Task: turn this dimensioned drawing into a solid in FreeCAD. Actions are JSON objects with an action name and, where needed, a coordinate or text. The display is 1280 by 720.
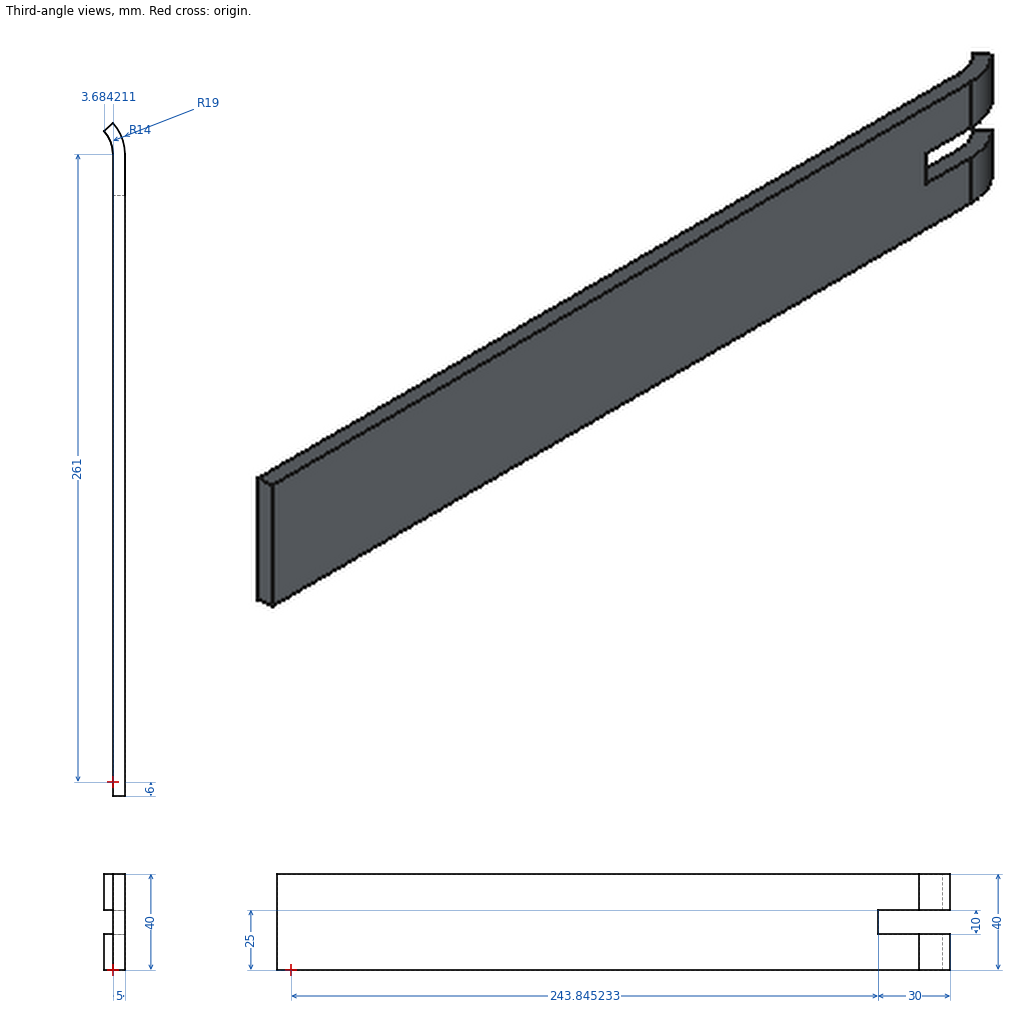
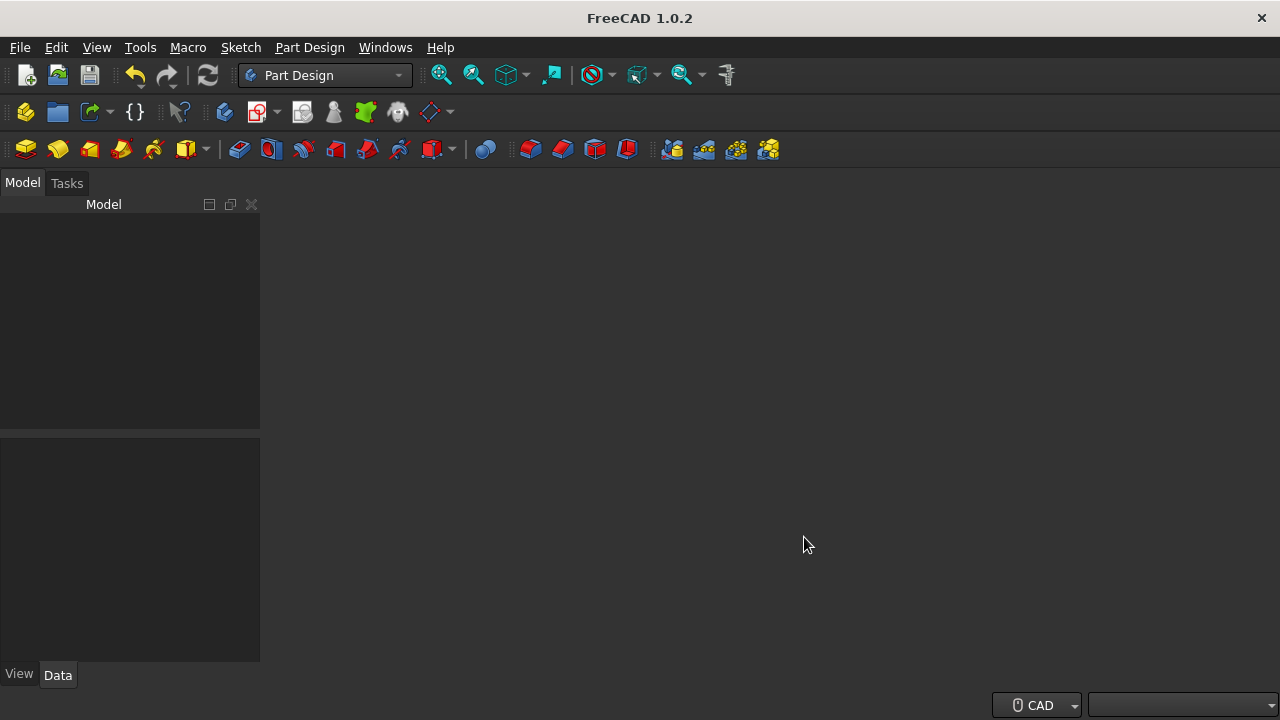
{"action": "left_click", "coordinate": [26, 76]}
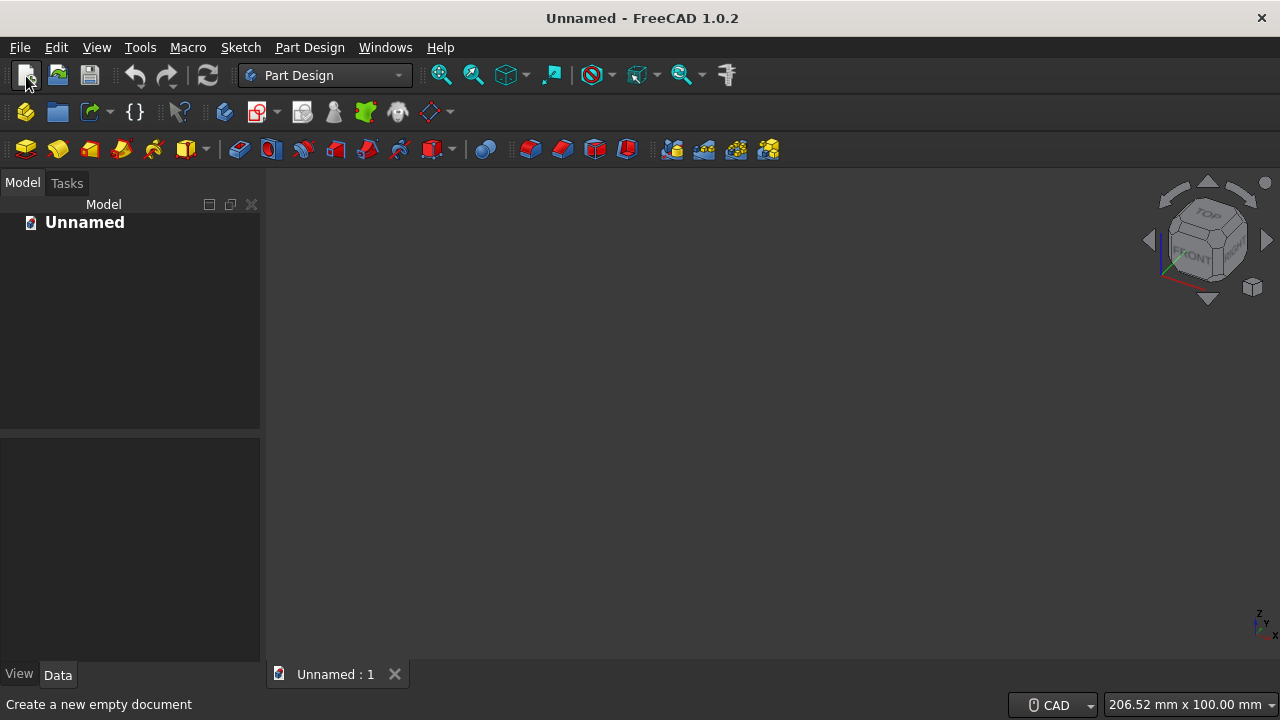
{"action": "left_click", "coordinate": [258, 112]}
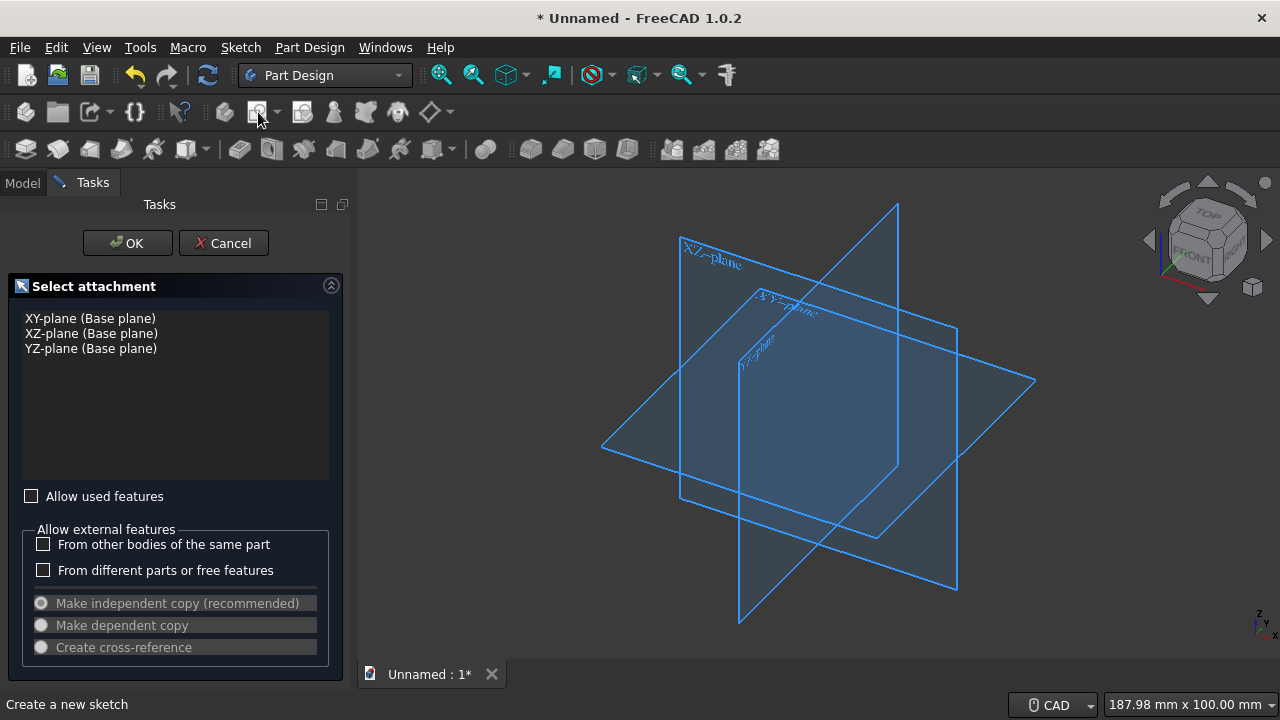
{"action": "left_click", "coordinate": [82, 318]}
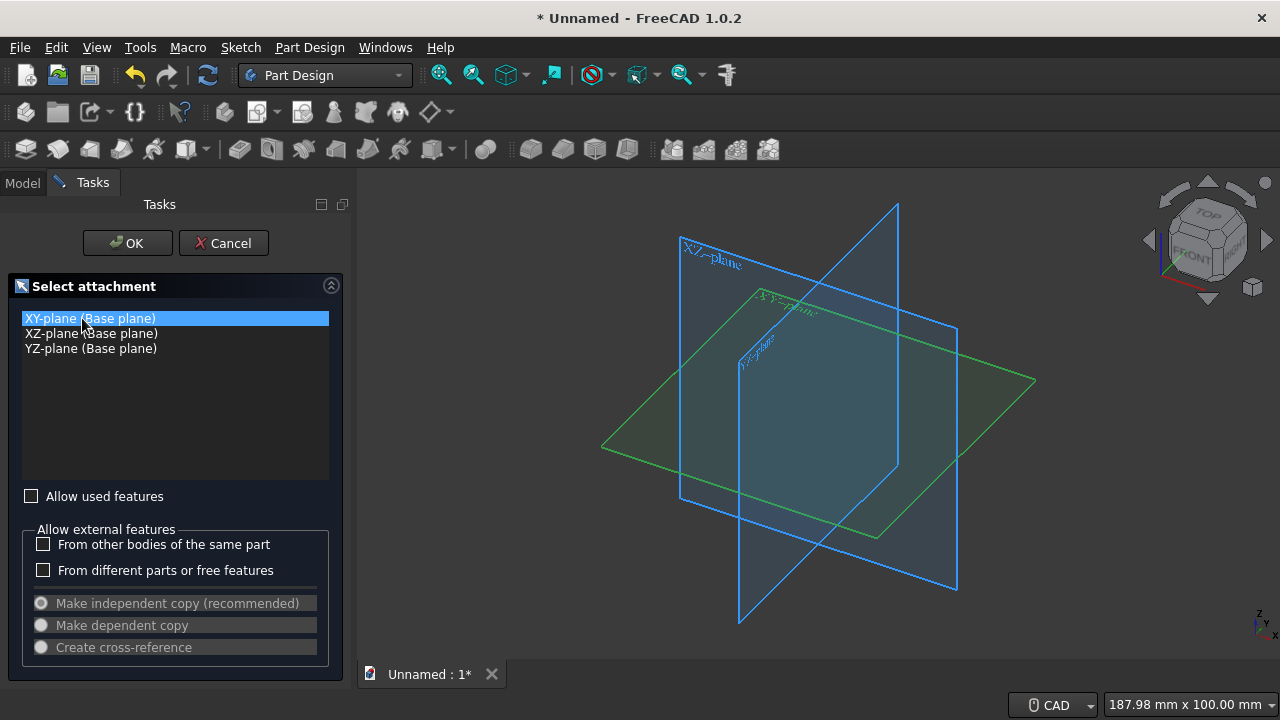
{"action": "left_click", "coordinate": [128, 243]}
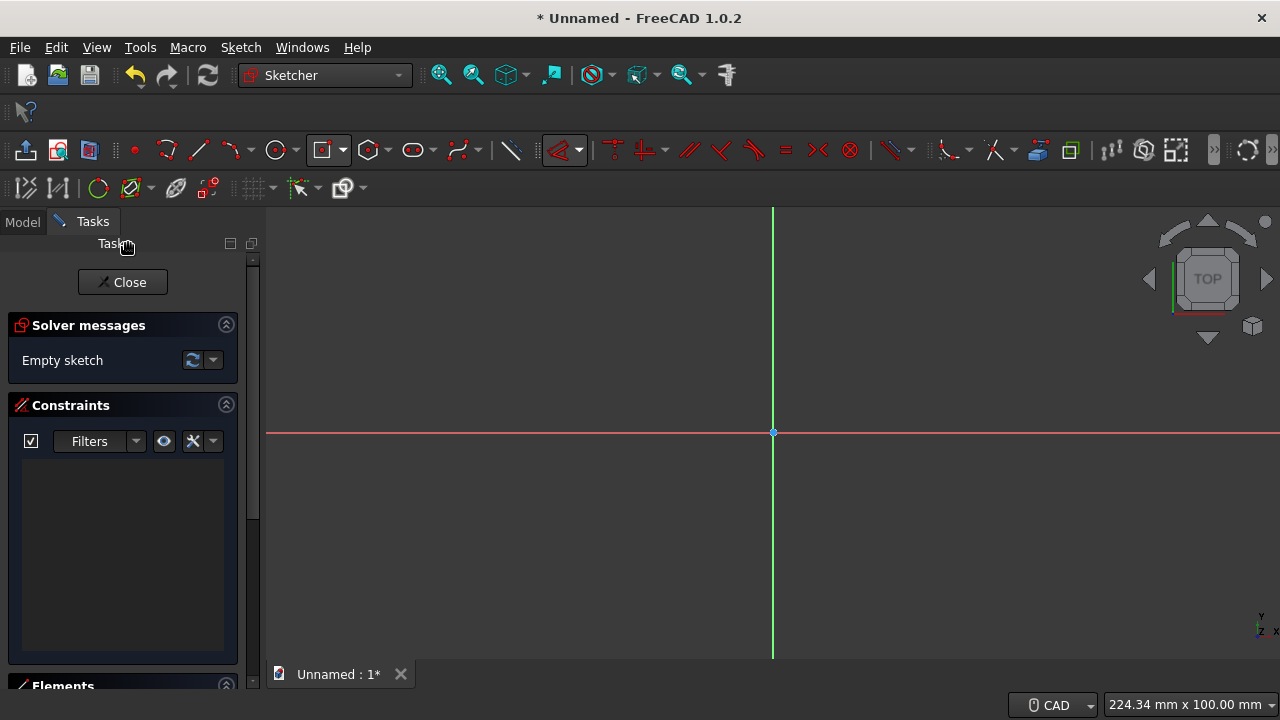
{"action": "scroll", "coordinate": [681, 631], "scroll_direction": "down", "scroll_amount": 7}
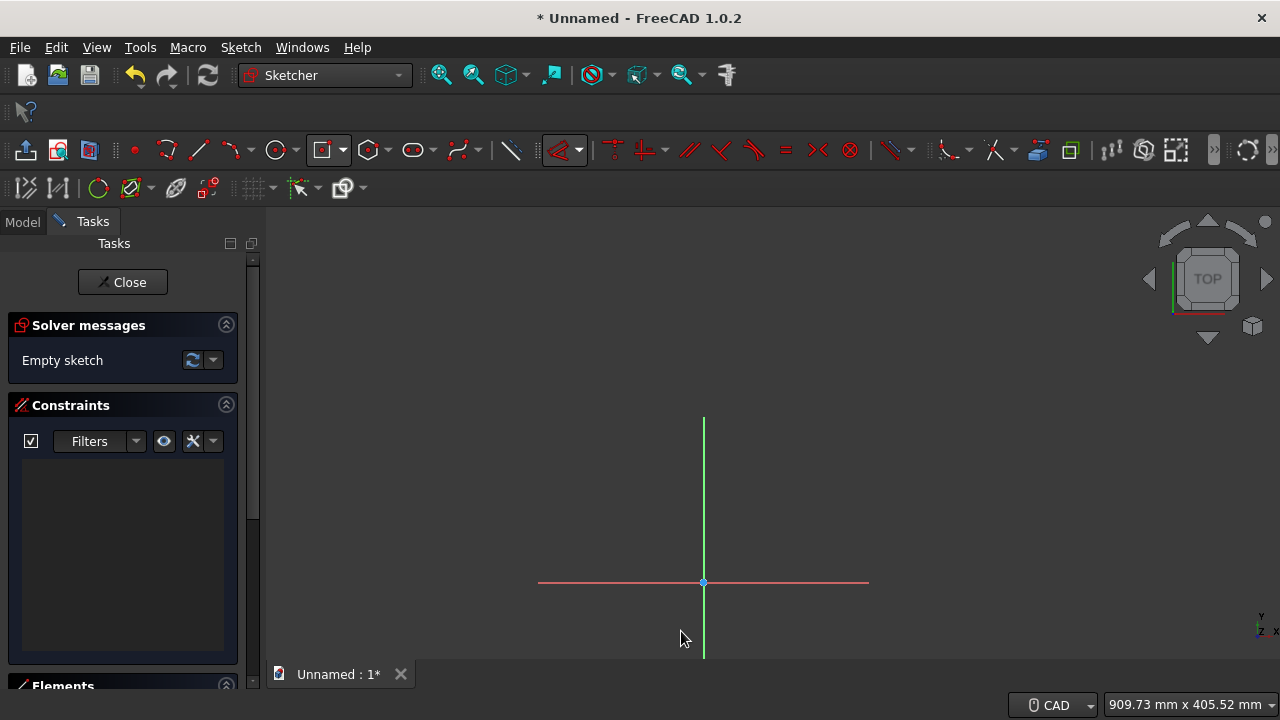
{"action": "left_click", "coordinate": [200, 150]}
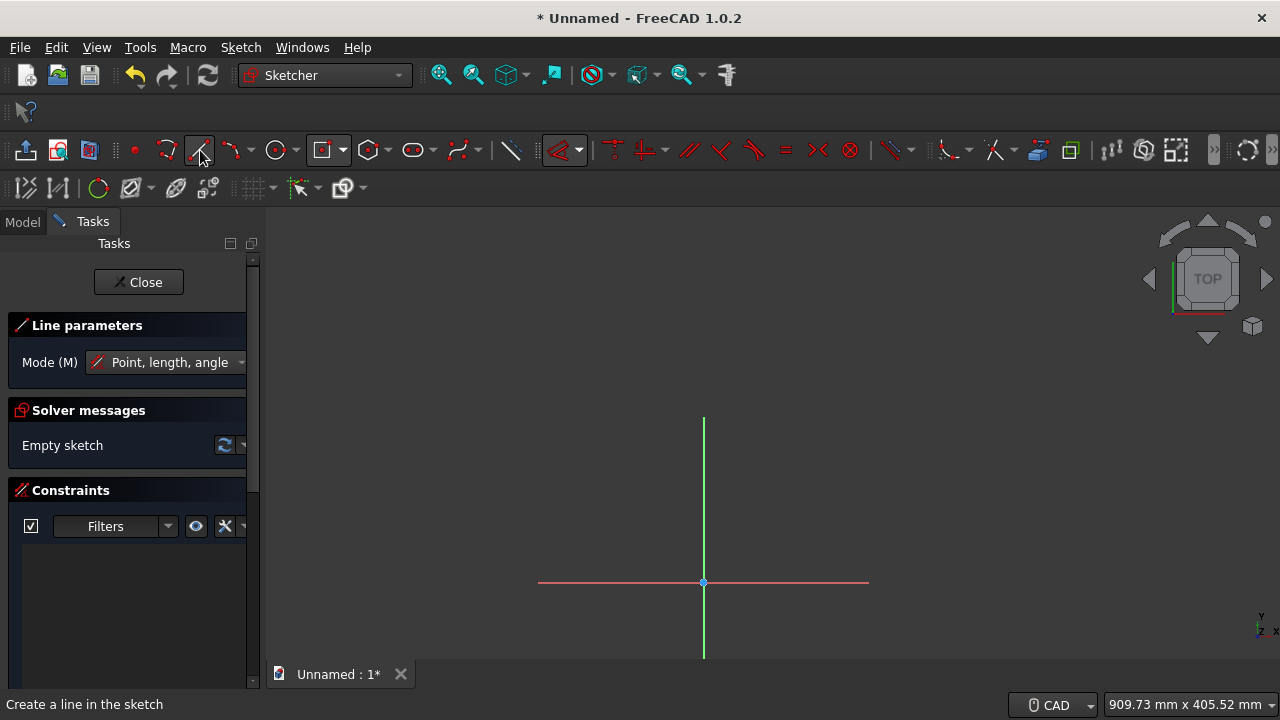
{"action": "left_click", "coordinate": [704, 278]}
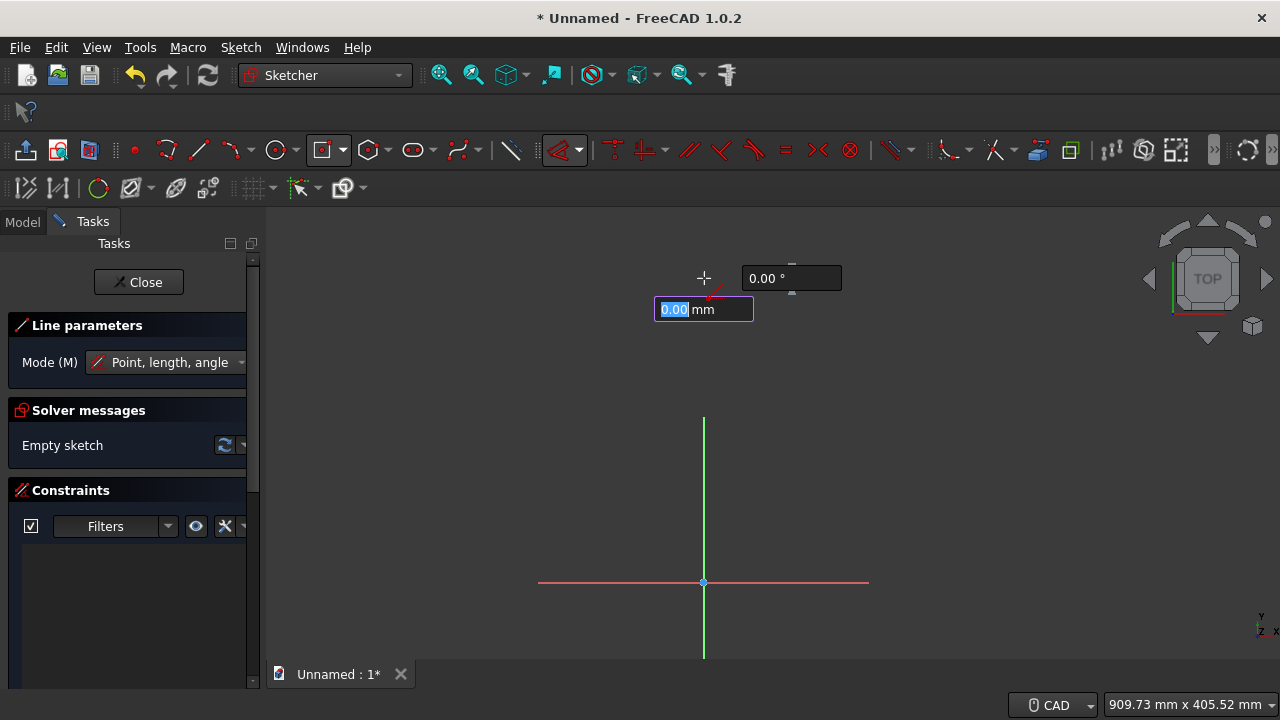
{"action": "scroll", "coordinate": [700, 281], "scroll_direction": "up", "scroll_amount": 7}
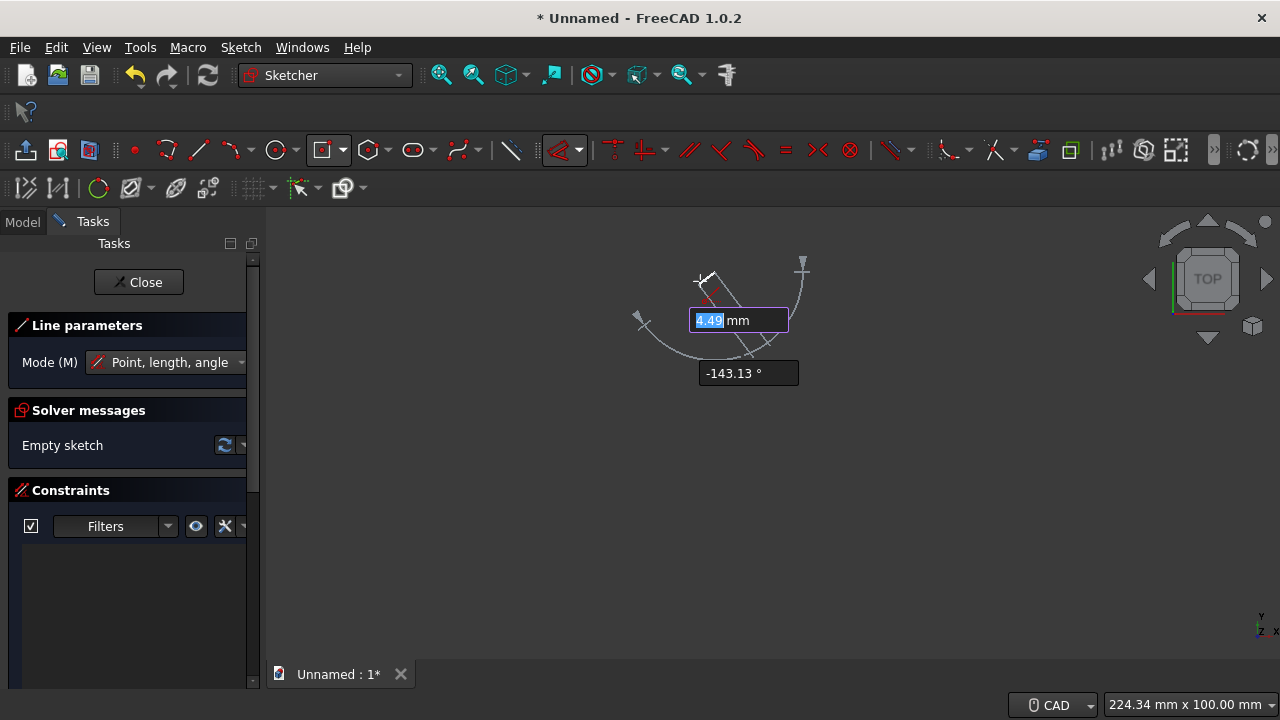
{"action": "left_click", "coordinate": [698, 282]}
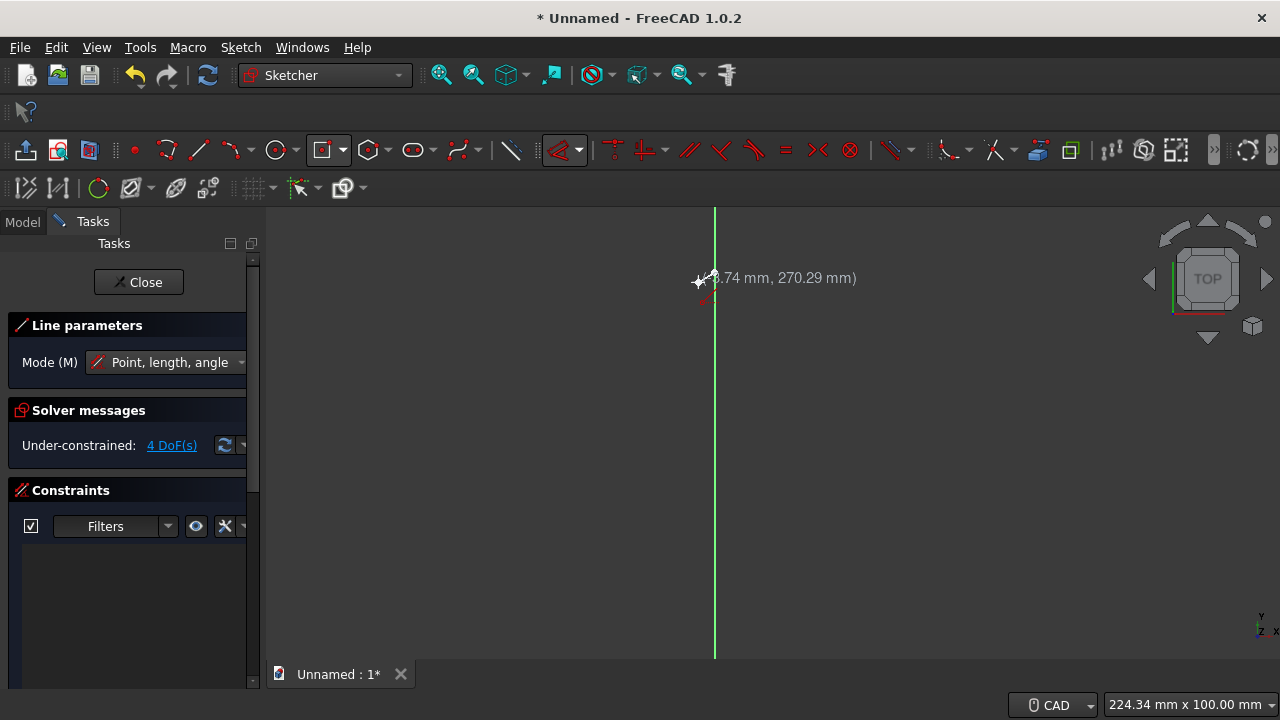
{"action": "left_click", "coordinate": [168, 150]}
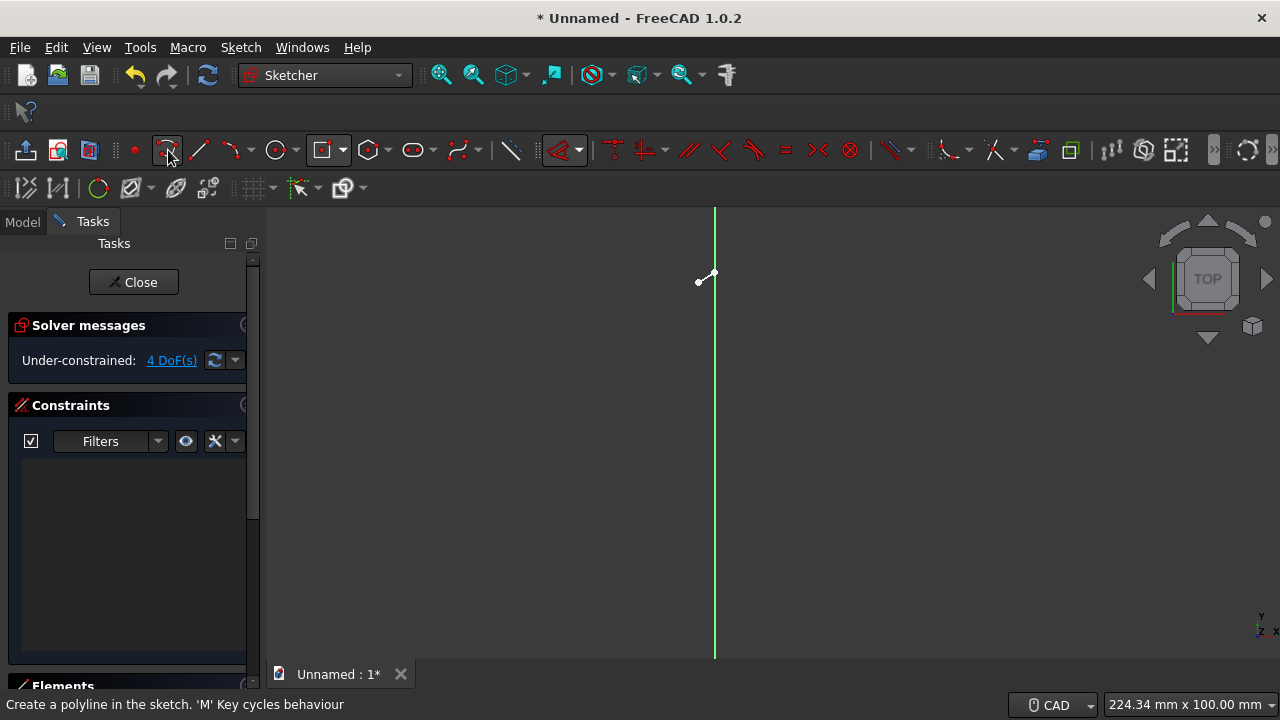
{"action": "scroll", "coordinate": [700, 285], "scroll_direction": "down", "scroll_amount": 7}